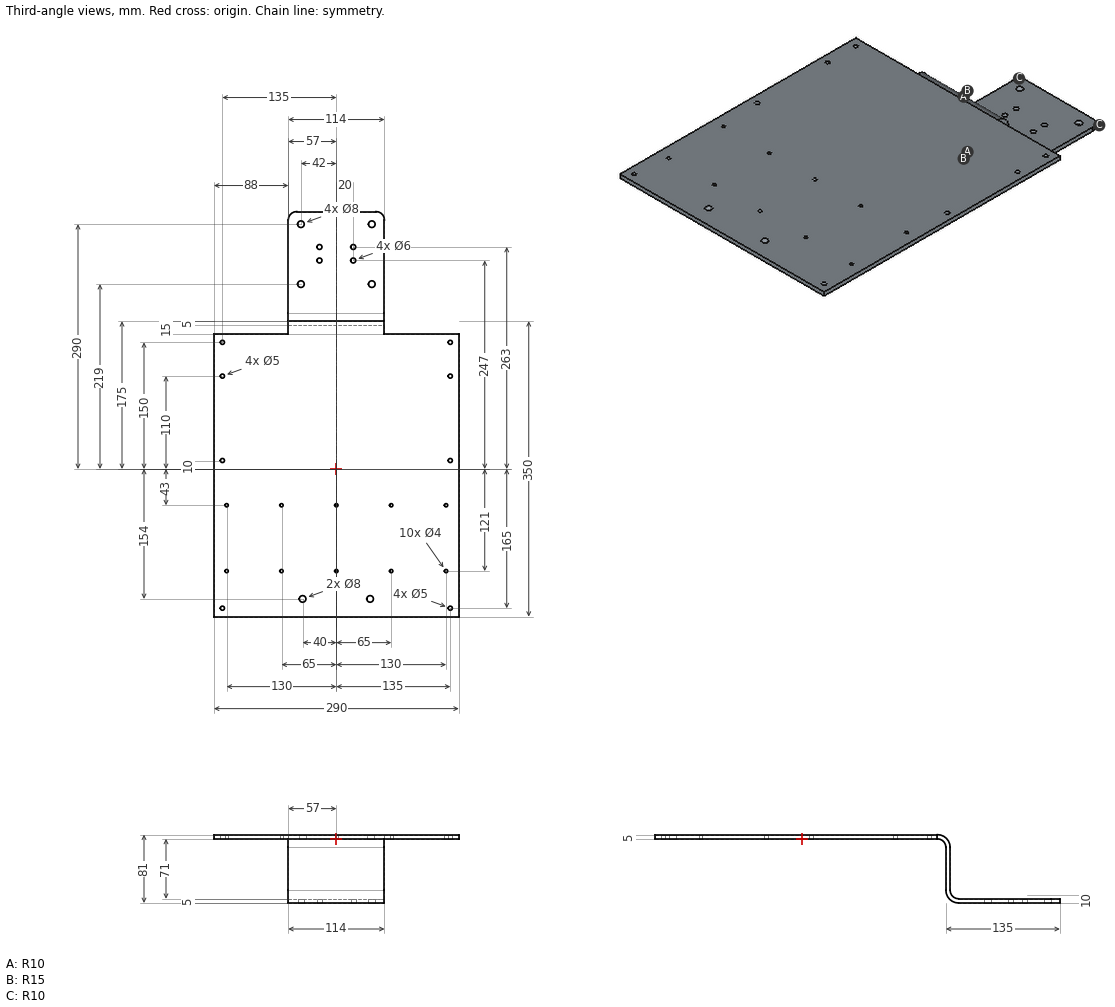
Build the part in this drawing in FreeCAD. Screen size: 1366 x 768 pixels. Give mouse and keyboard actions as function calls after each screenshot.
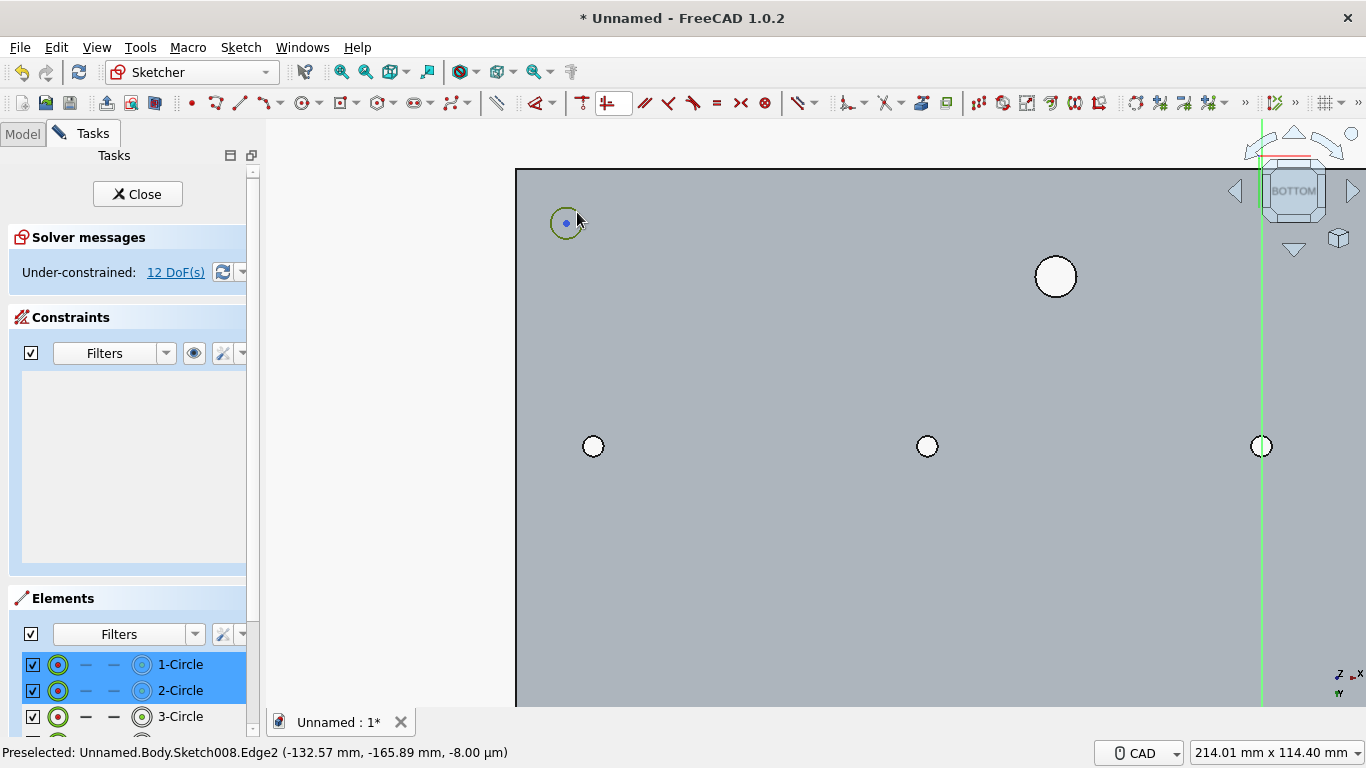
scroll(579, 211, down, 7)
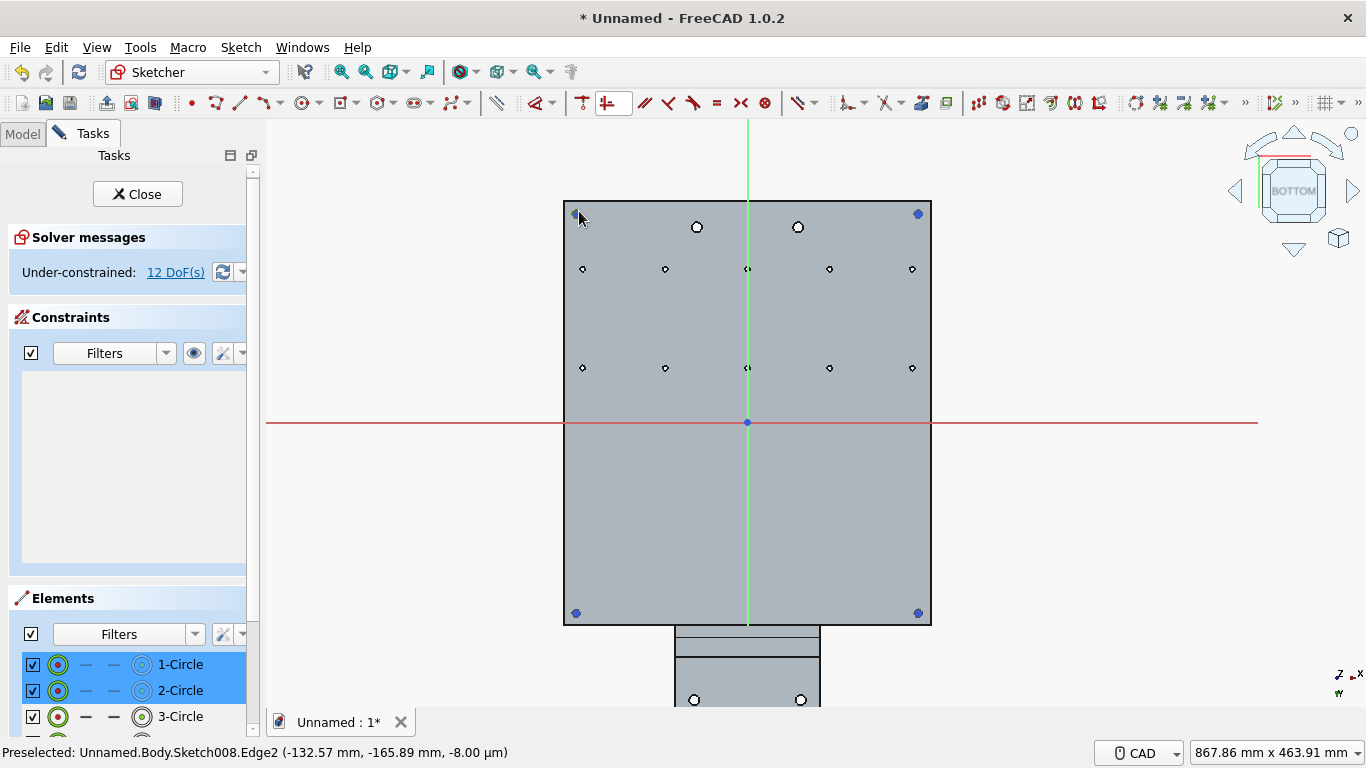
scroll(579, 611, up, 7)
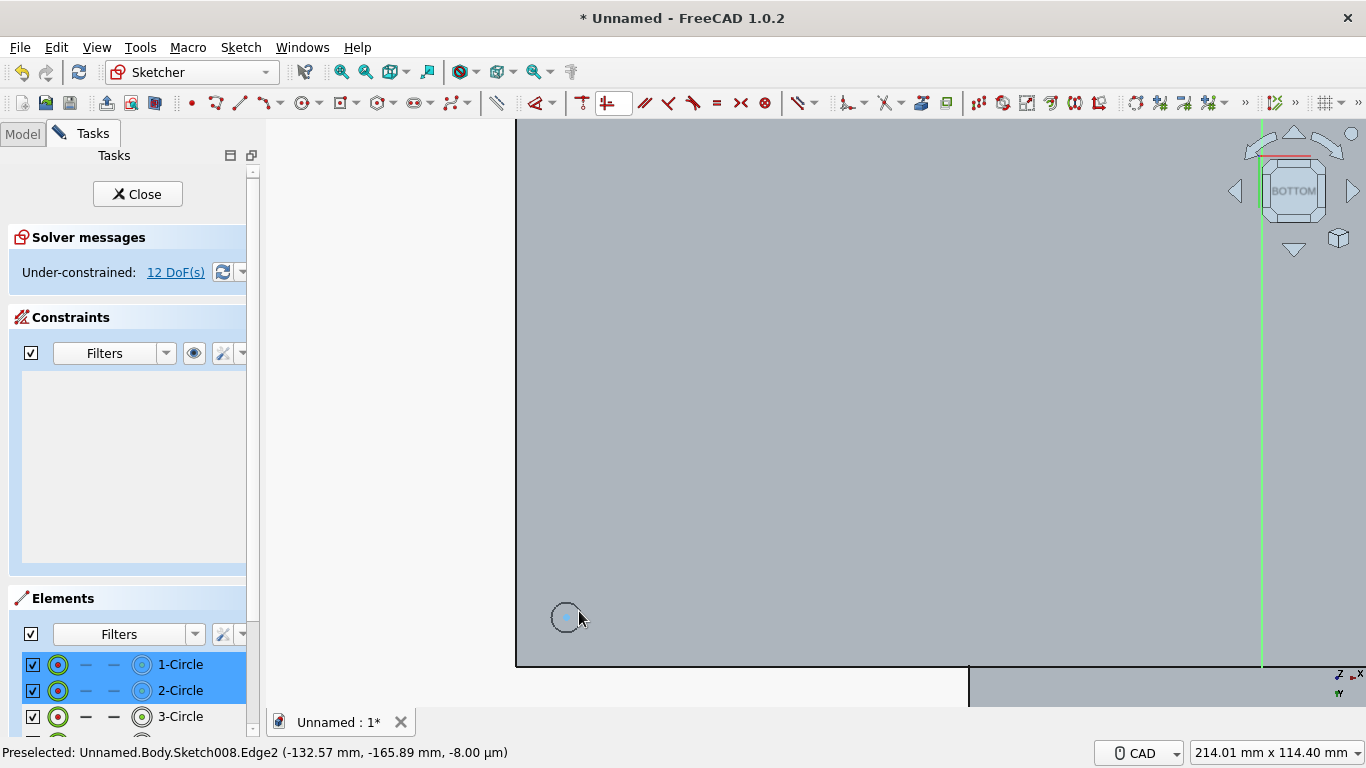
click(577, 607)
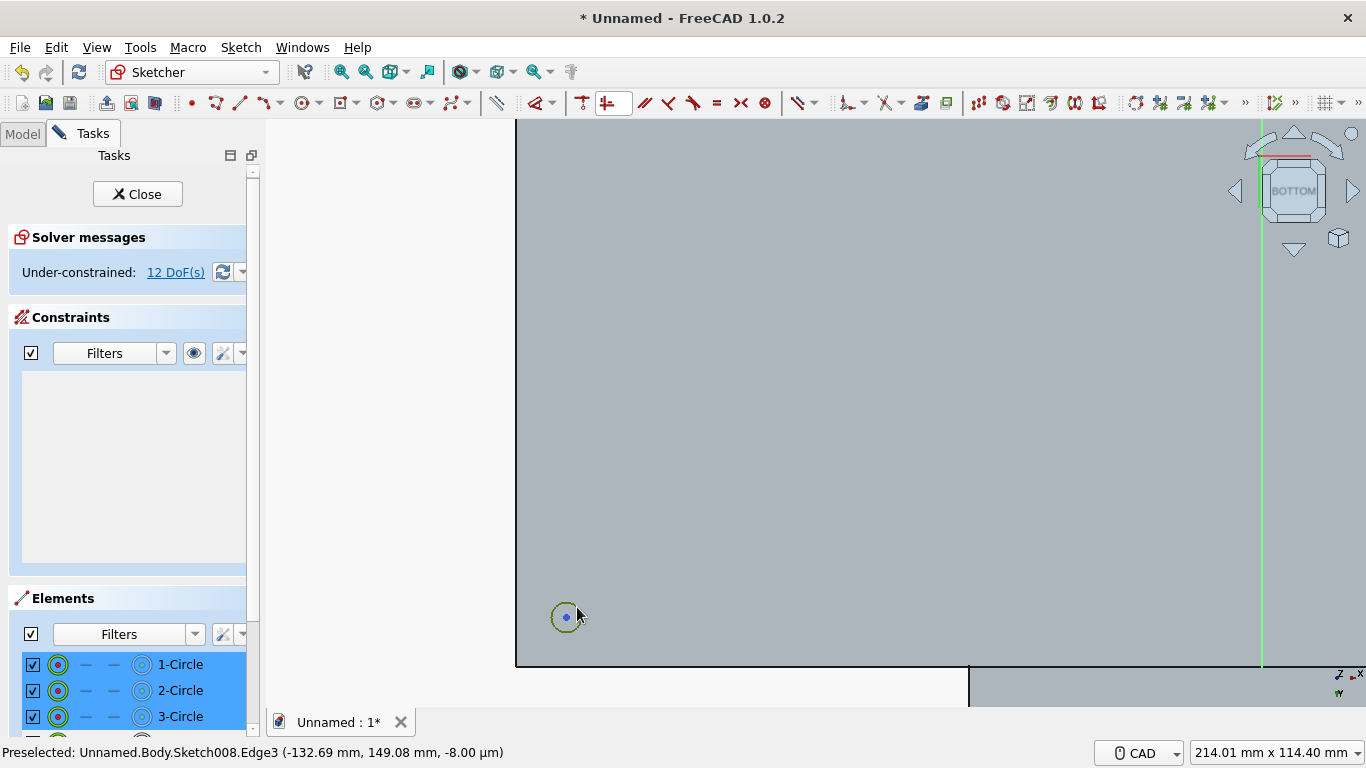
scroll(579, 612, down, 7)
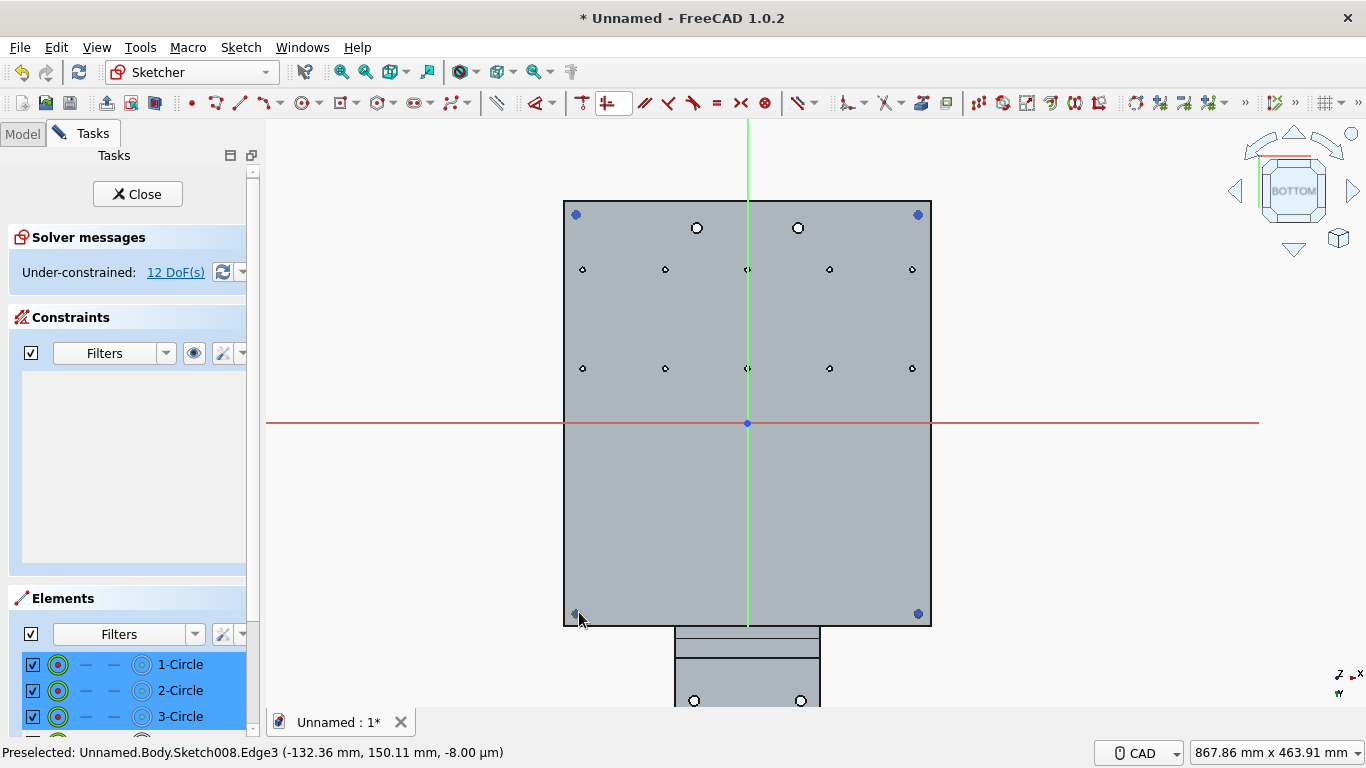
scroll(921, 611, up, 7)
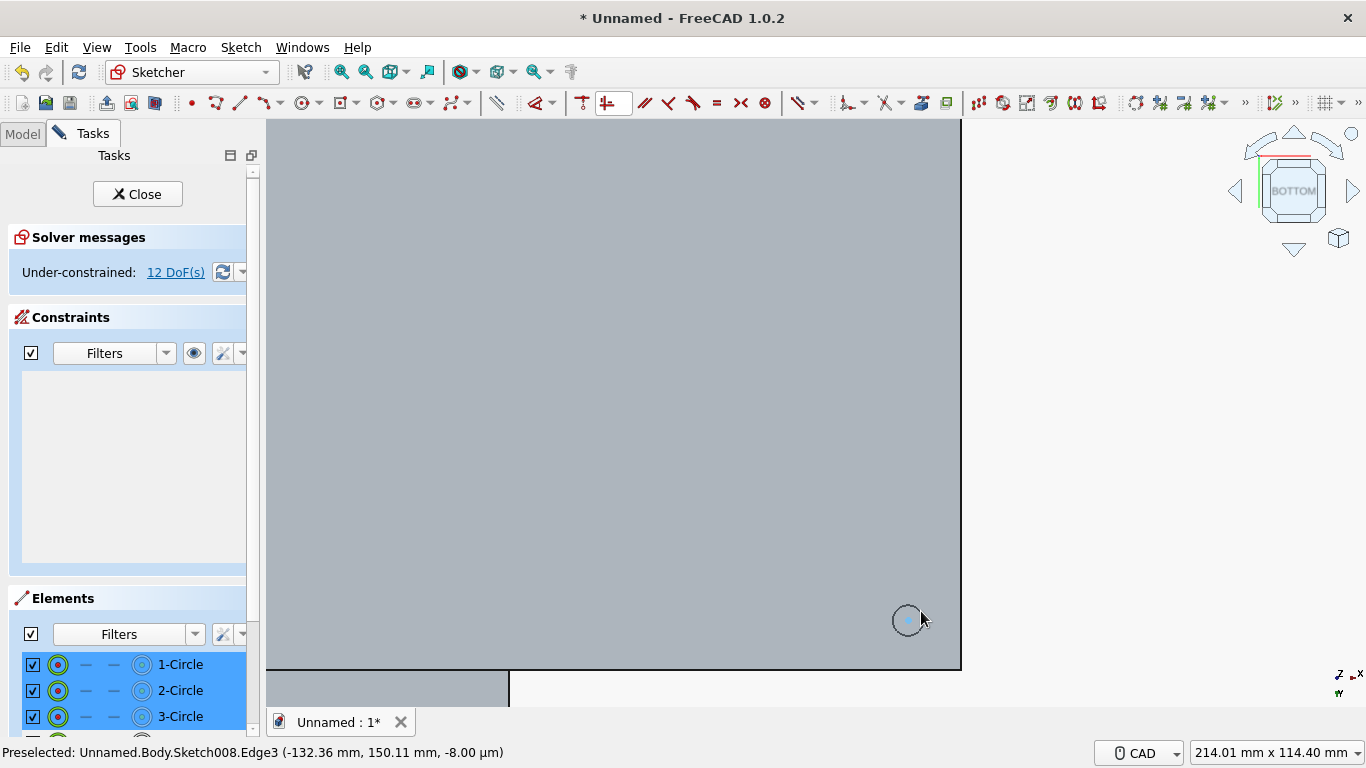
click(919, 610)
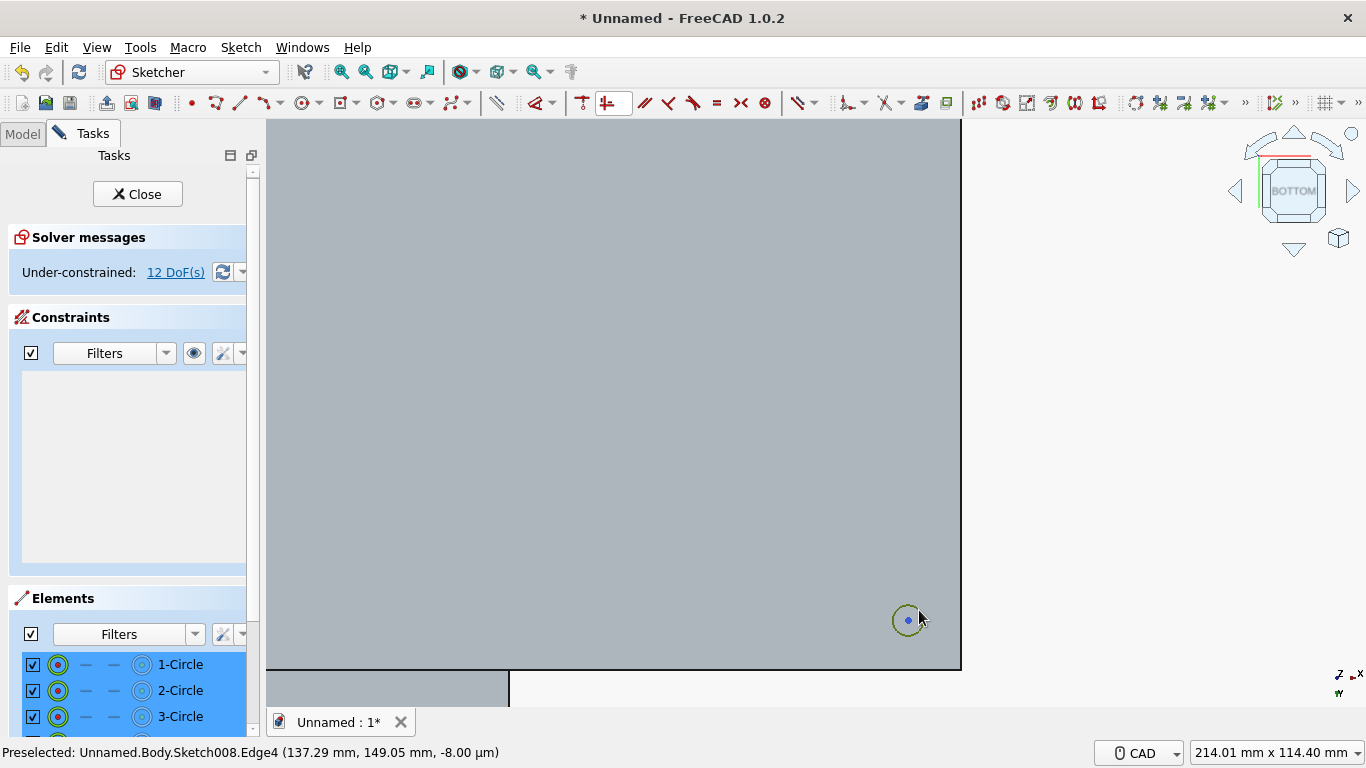
click(718, 104)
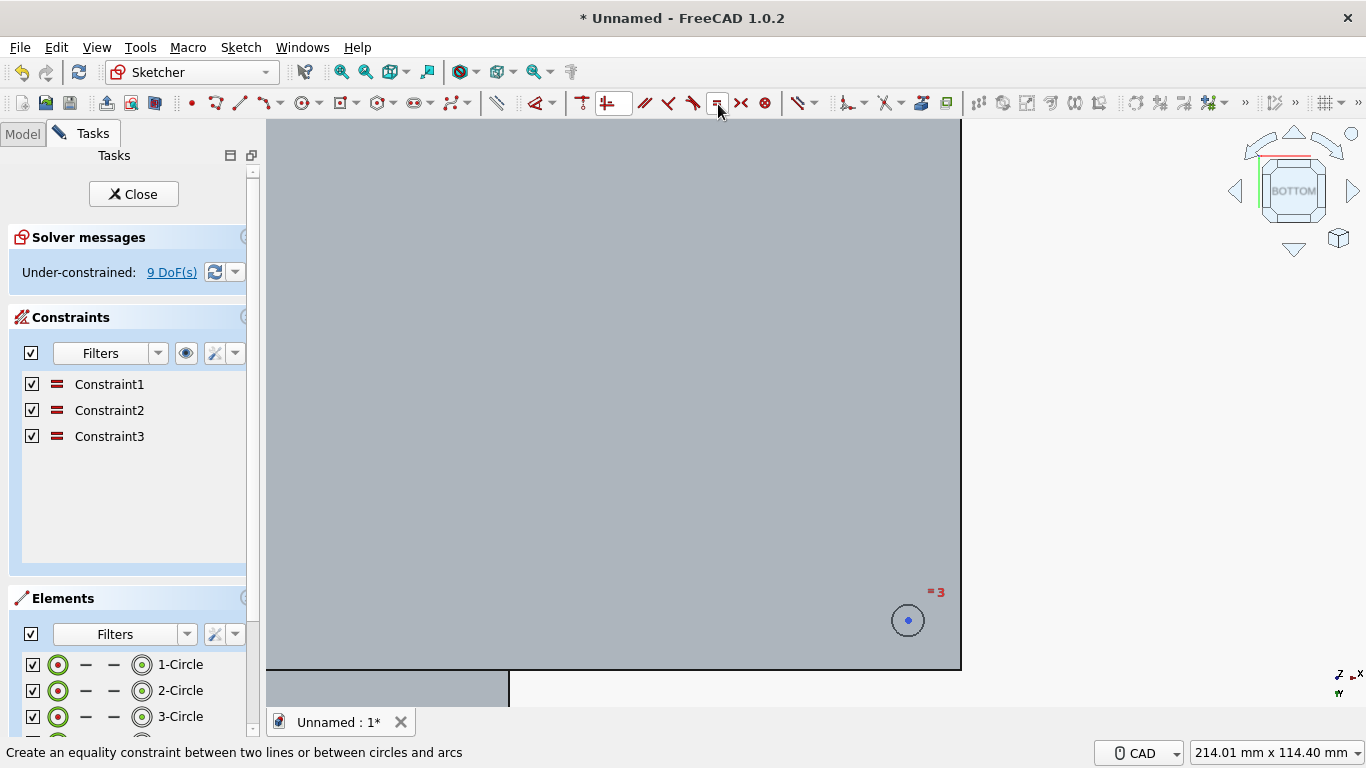
scroll(922, 611, down, 7)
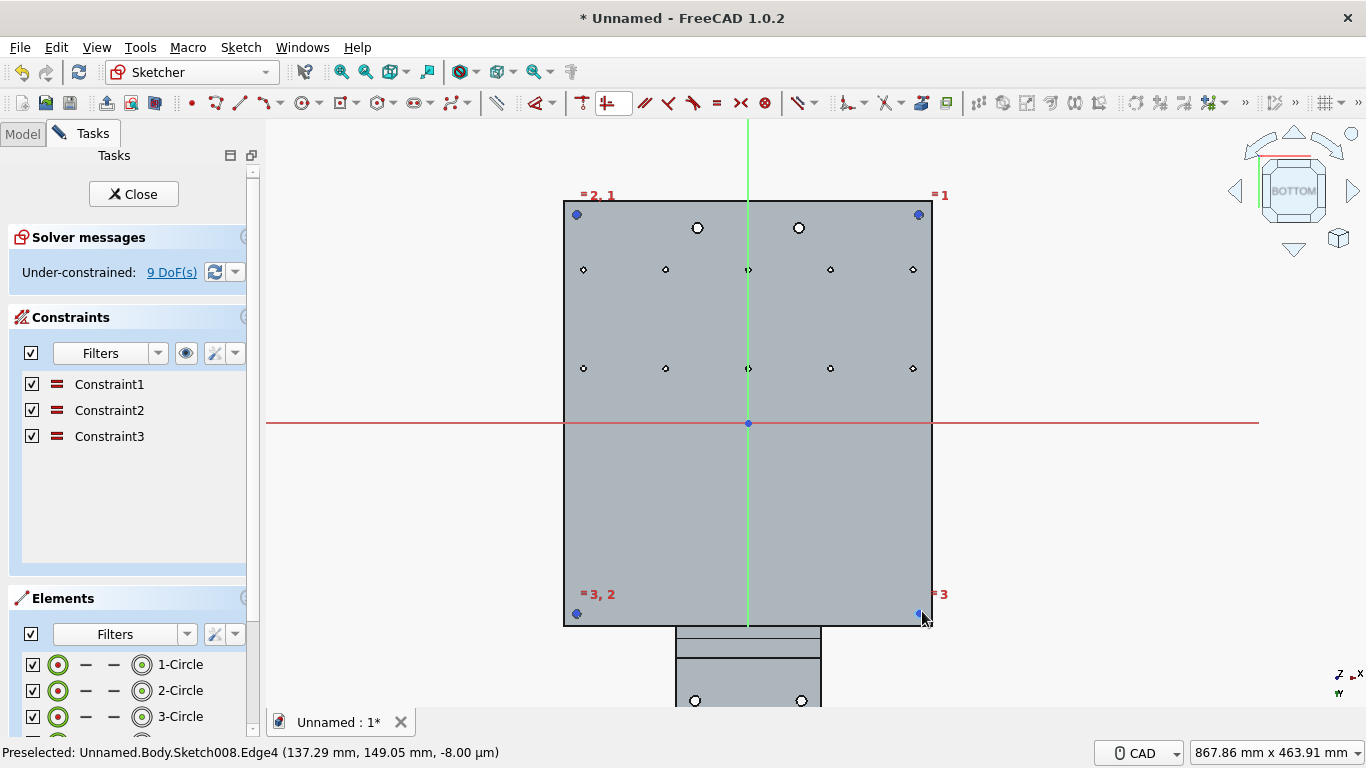
click(919, 215)